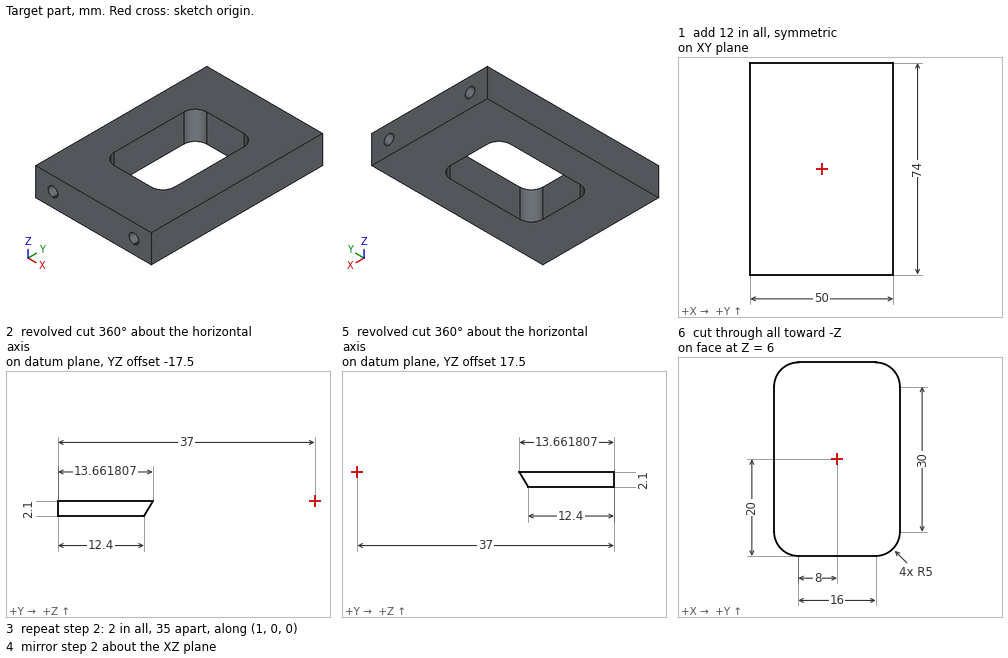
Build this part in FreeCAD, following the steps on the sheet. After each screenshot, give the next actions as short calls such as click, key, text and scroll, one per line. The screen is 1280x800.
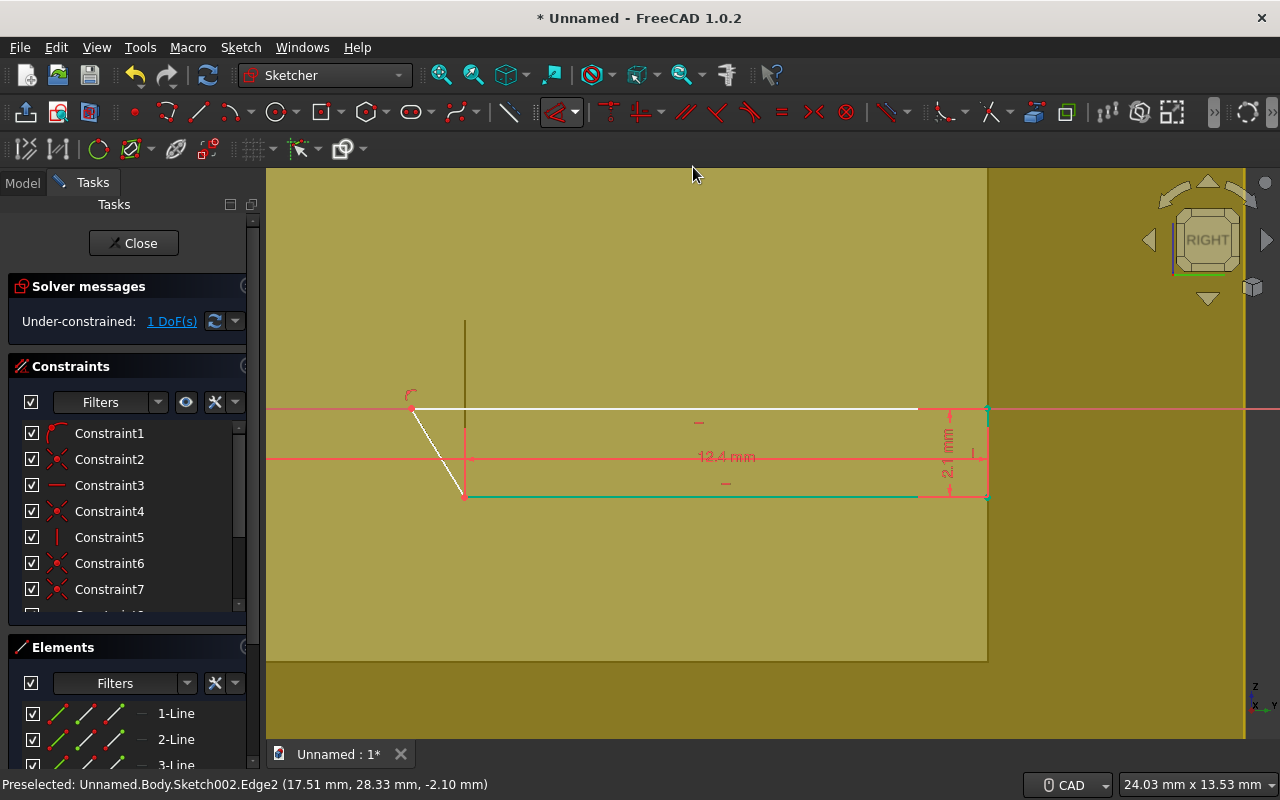
click(815, 409)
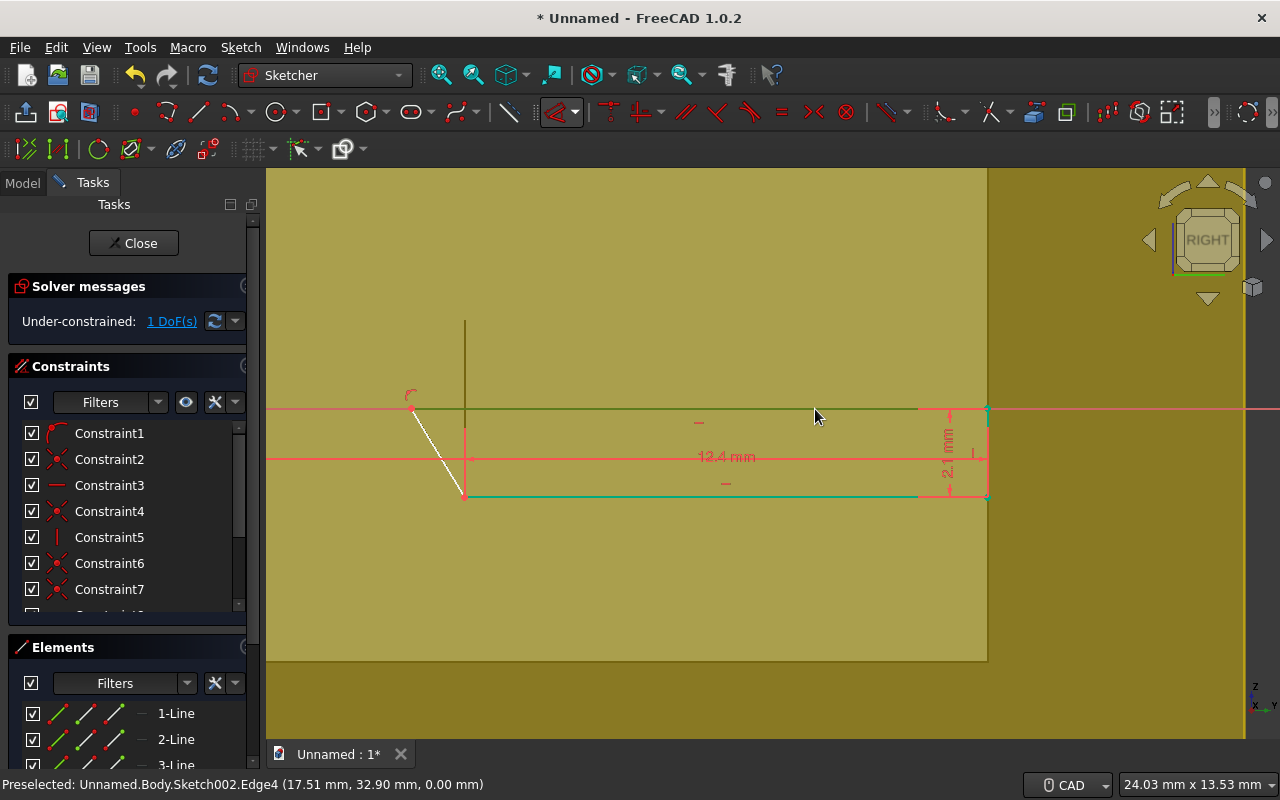
click(578, 112)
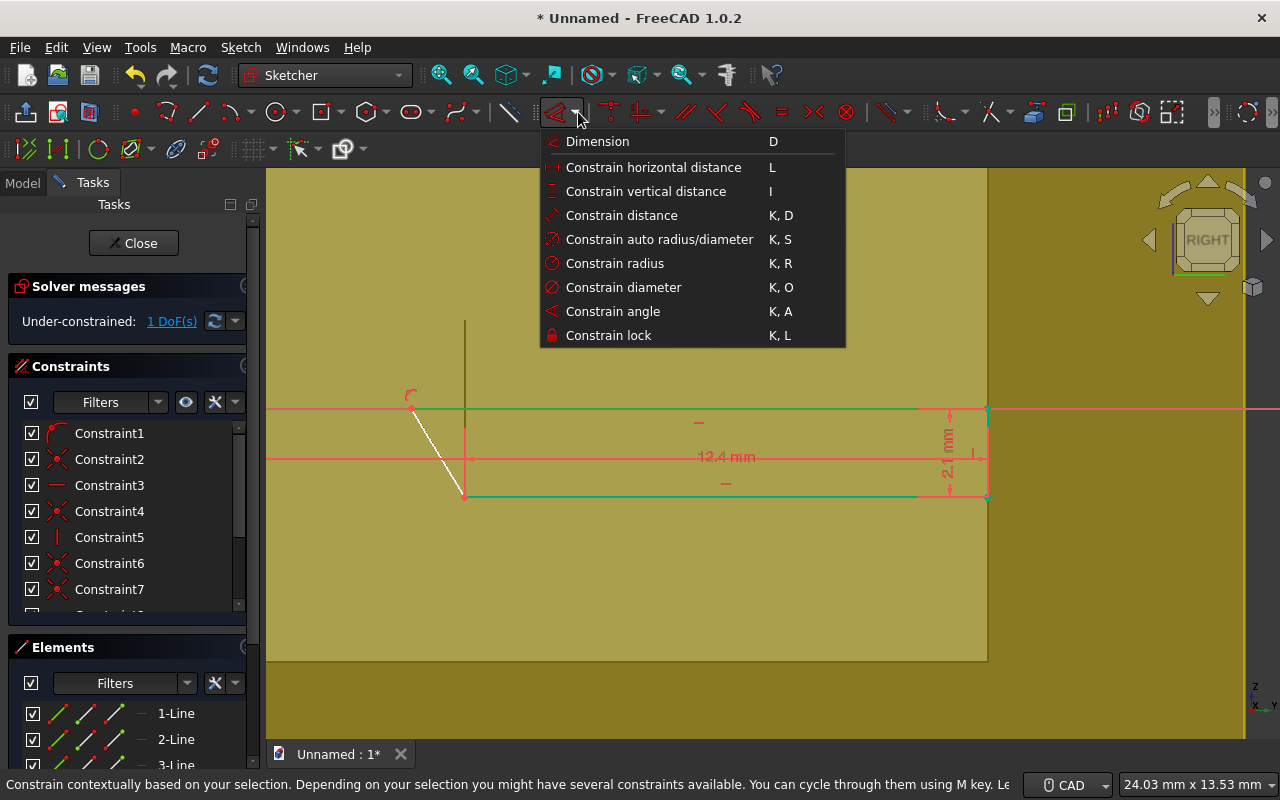
click(693, 167)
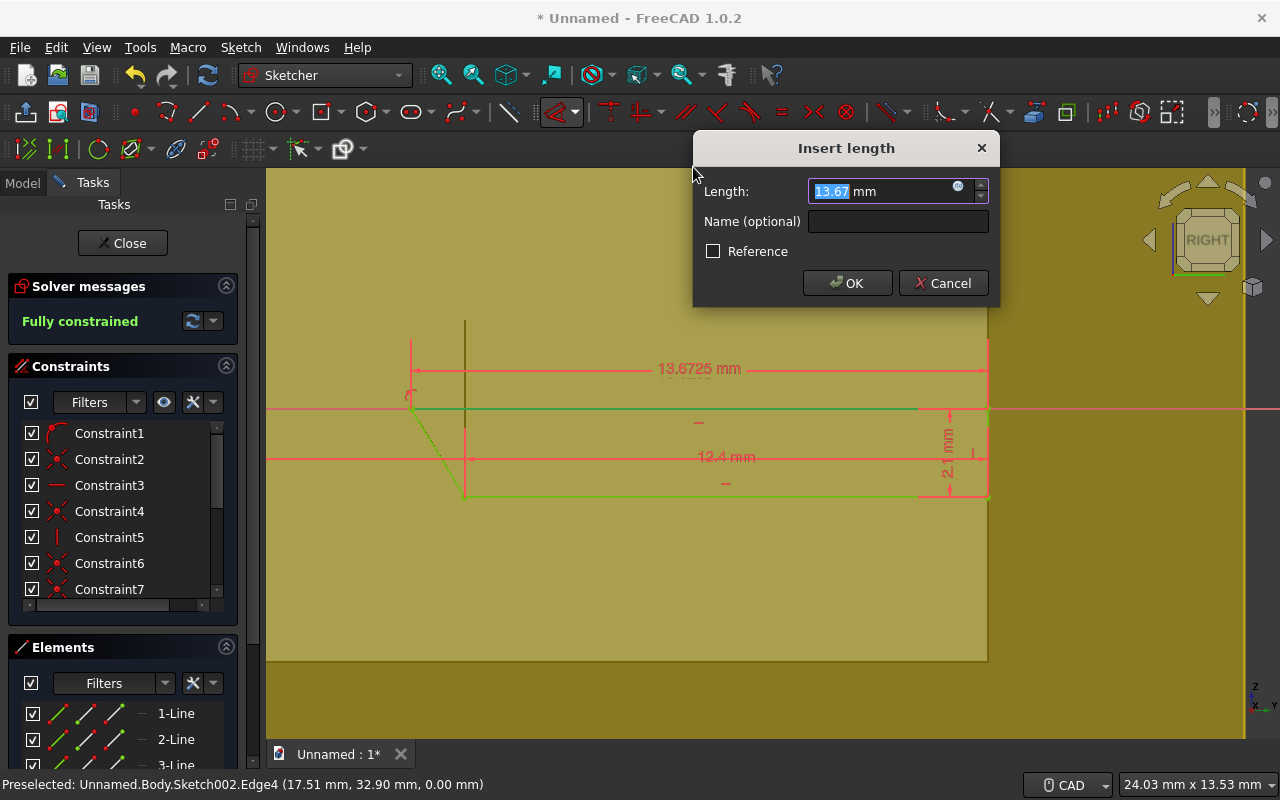
text(13.661807)
key(Return)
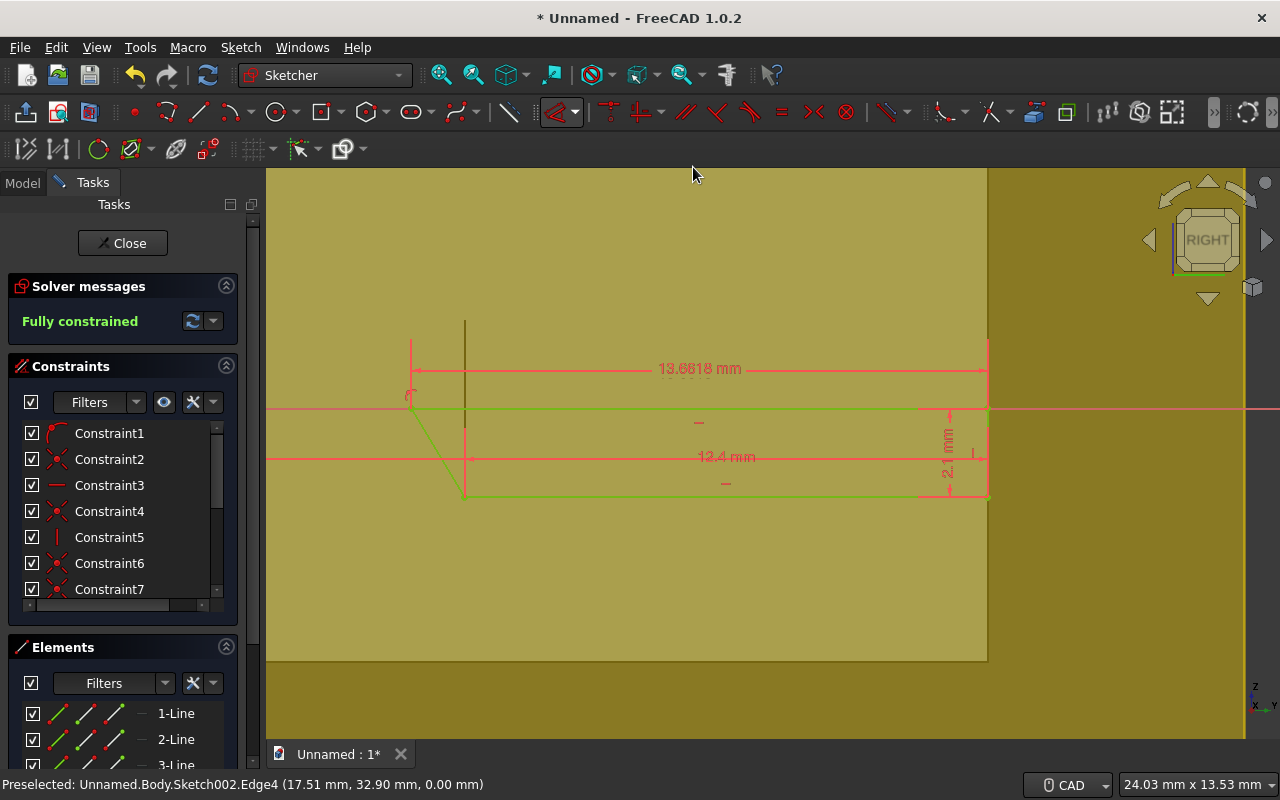
click(123, 243)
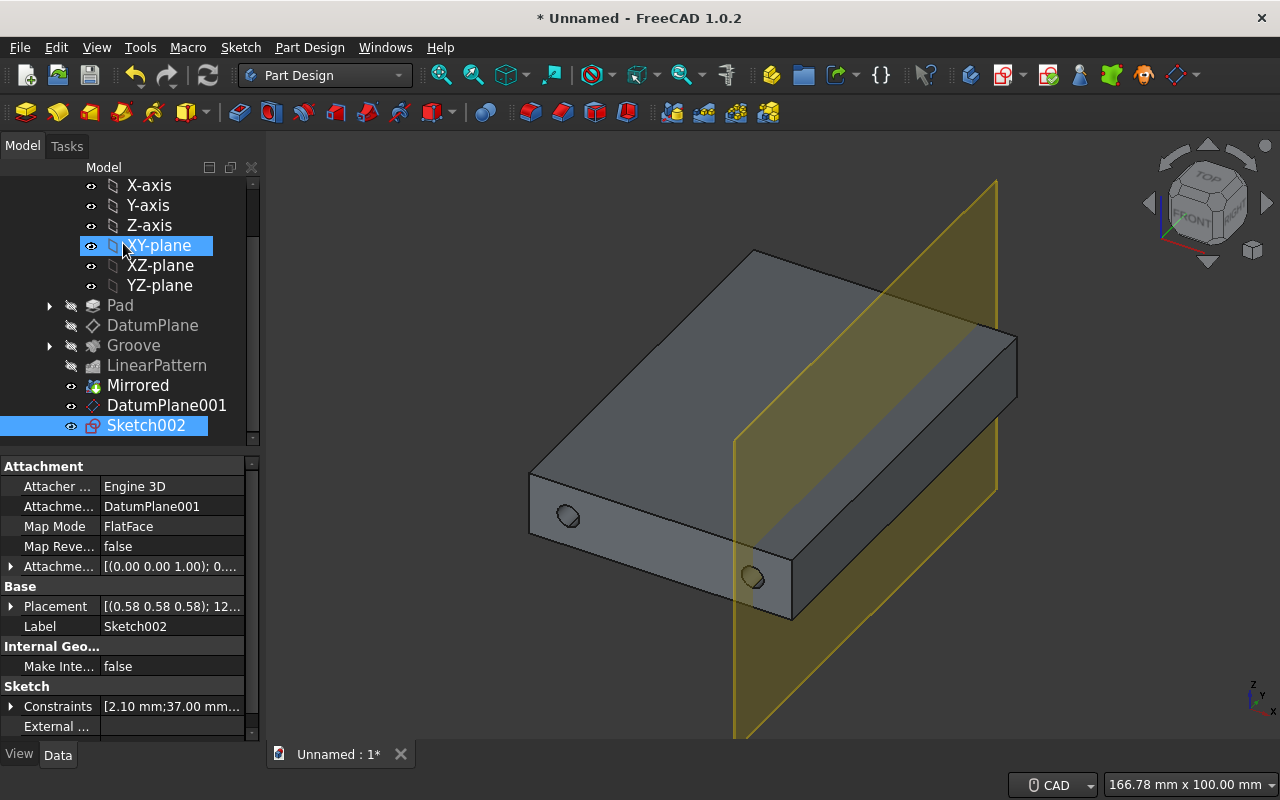
click(304, 112)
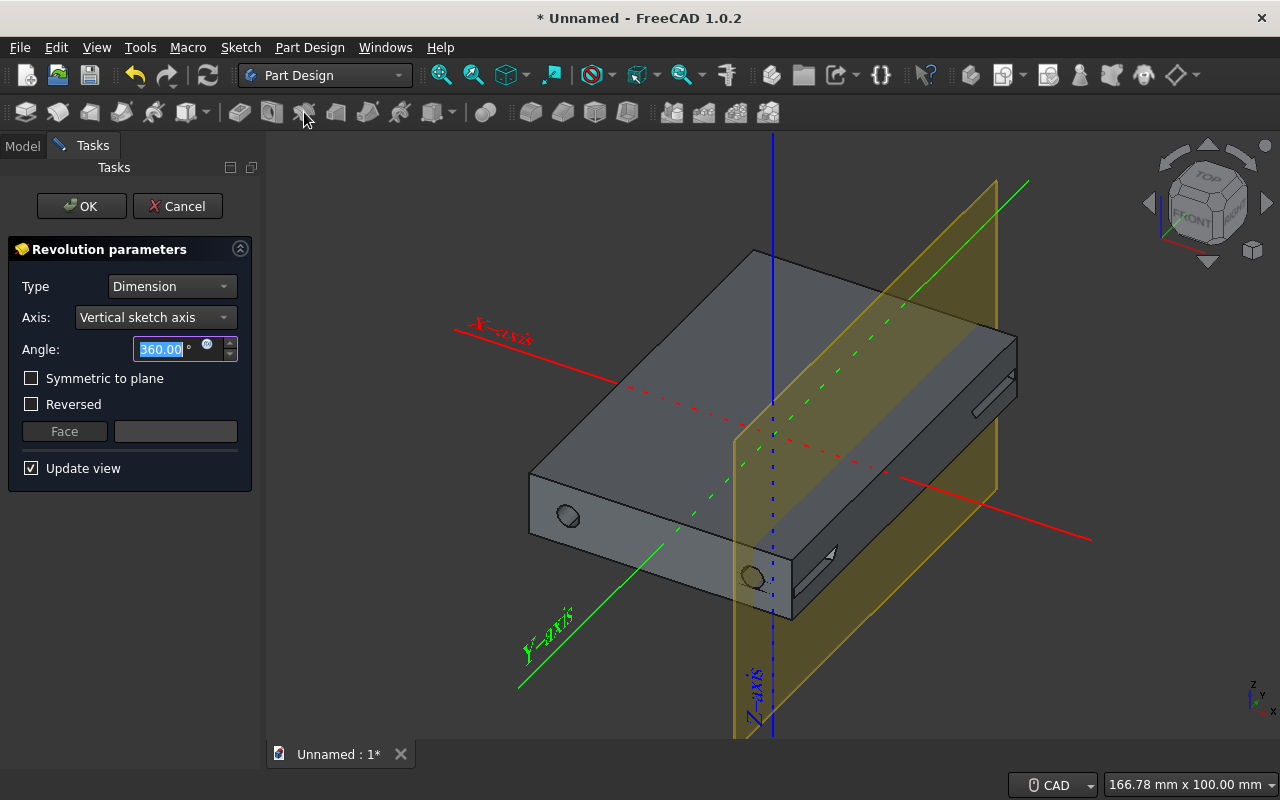
click(156, 318)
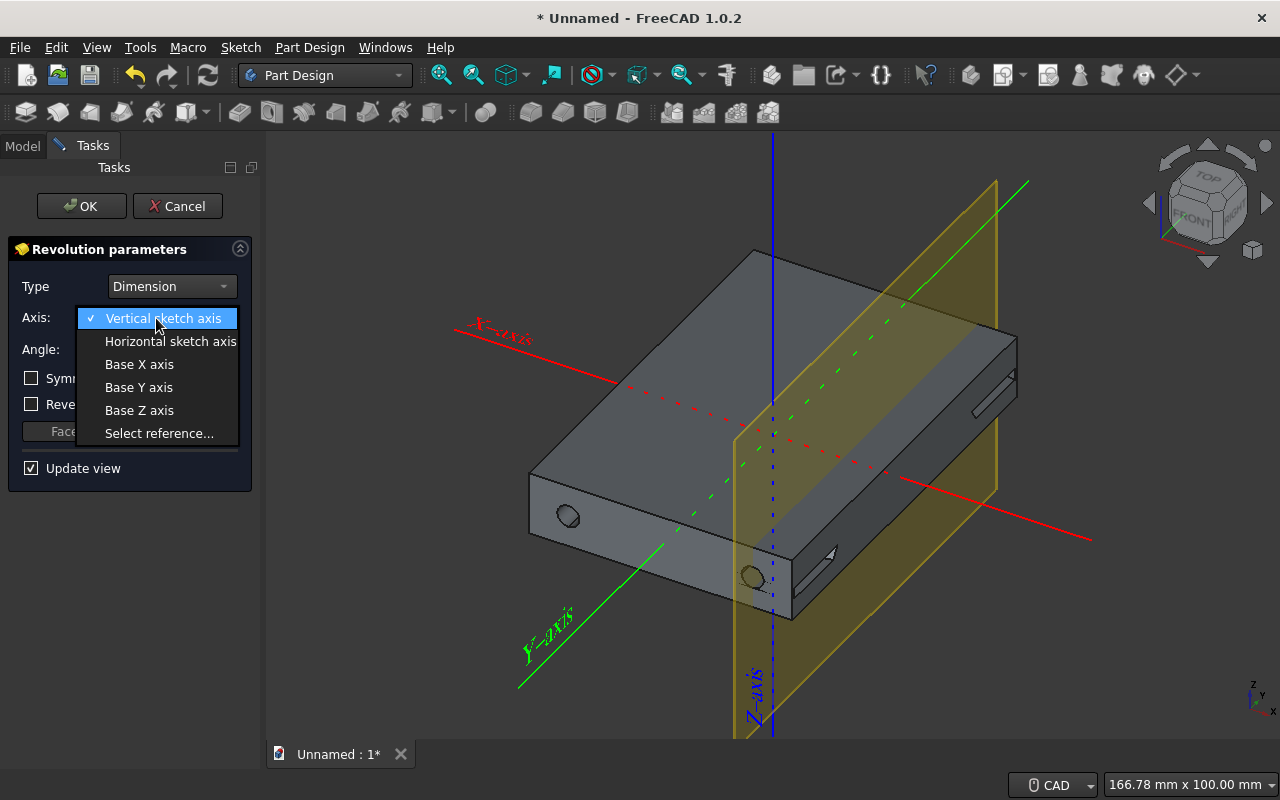
click(156, 342)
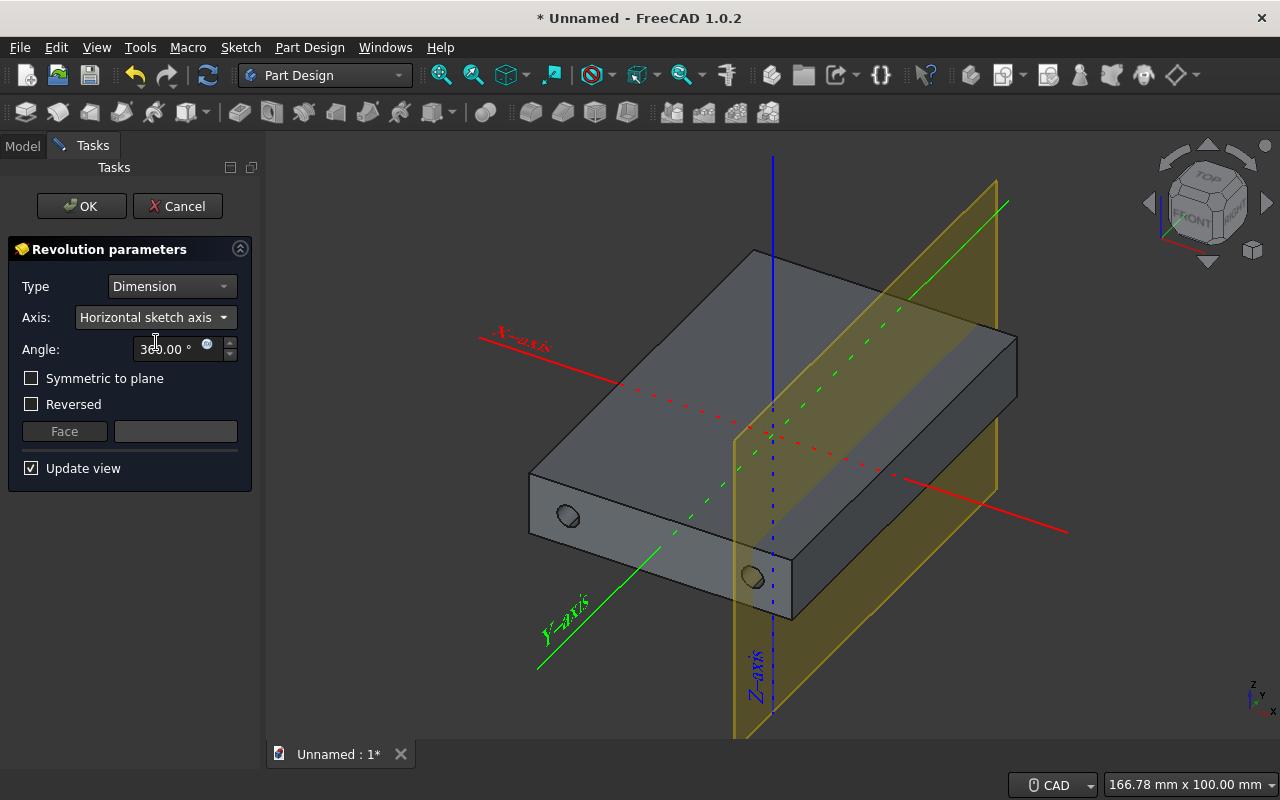
click(82, 206)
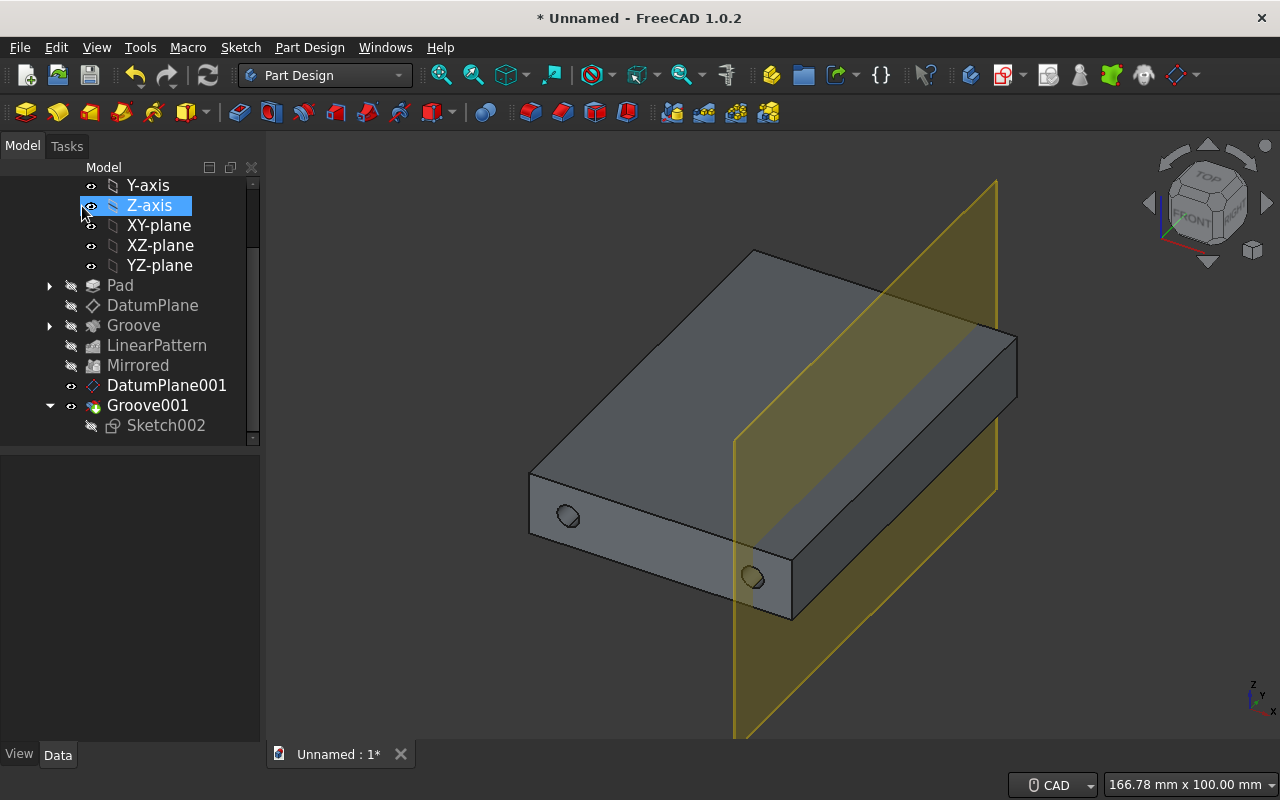
click(116, 386)
key(space)